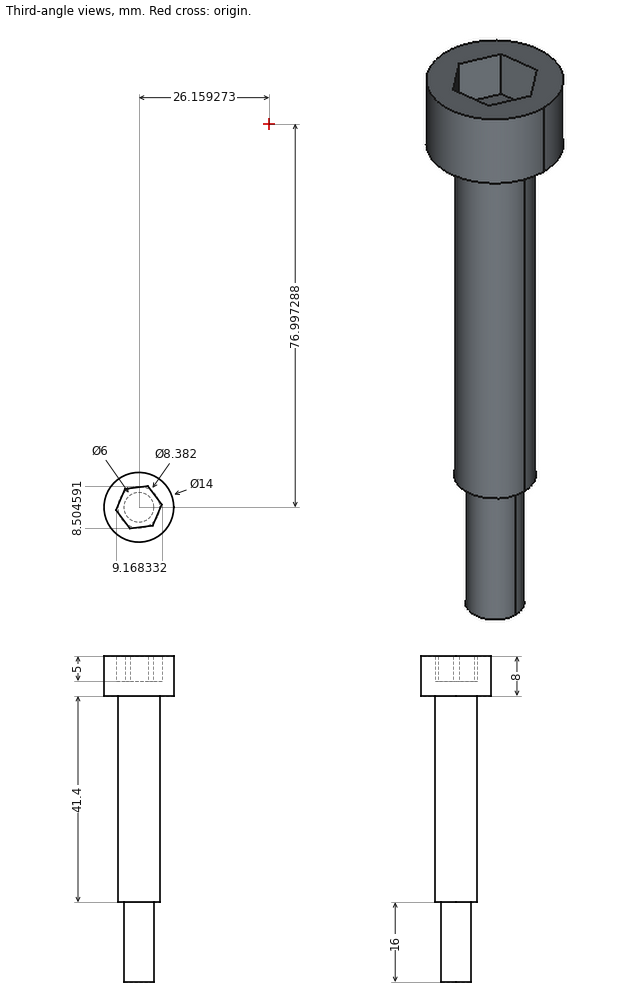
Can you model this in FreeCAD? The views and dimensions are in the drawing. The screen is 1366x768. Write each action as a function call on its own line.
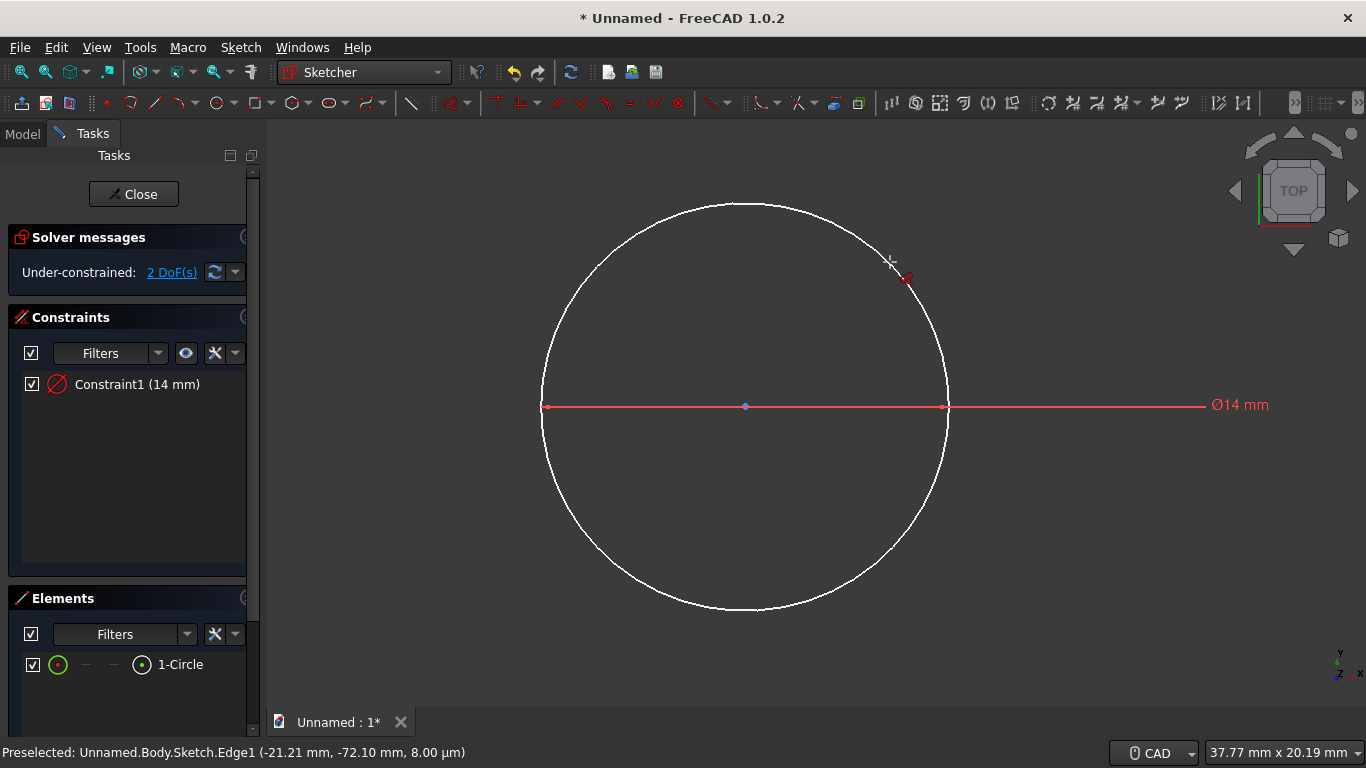
click(745, 407)
click(973, 441)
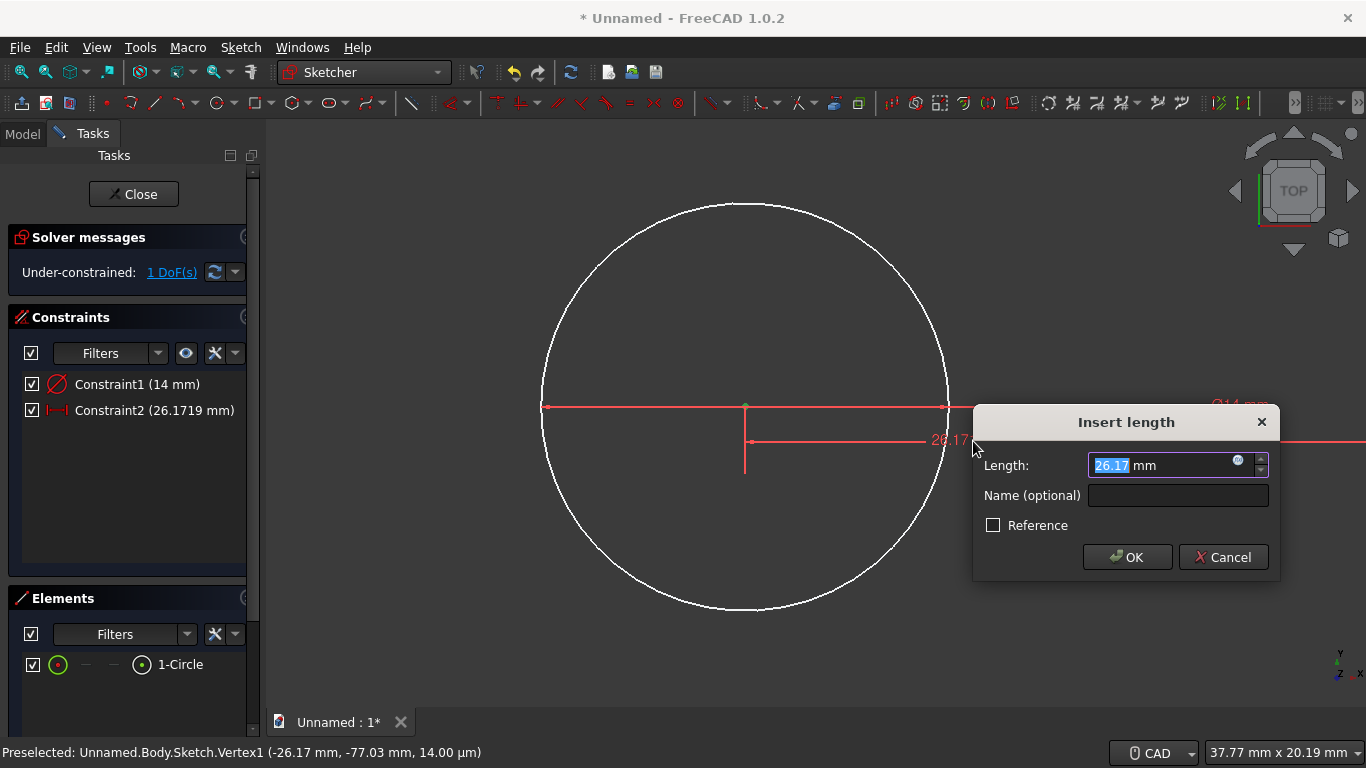
text(26.159273)
key(Return)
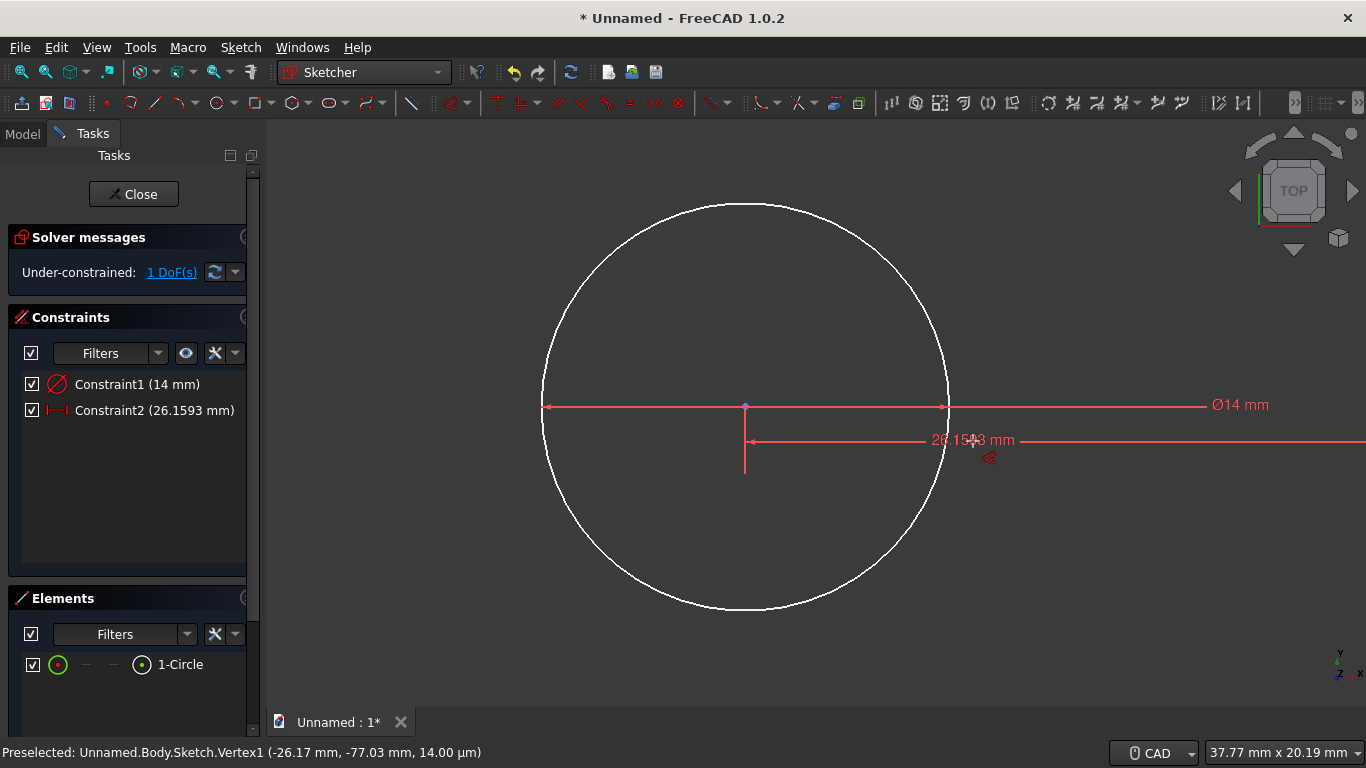
click(745, 407)
click(711, 277)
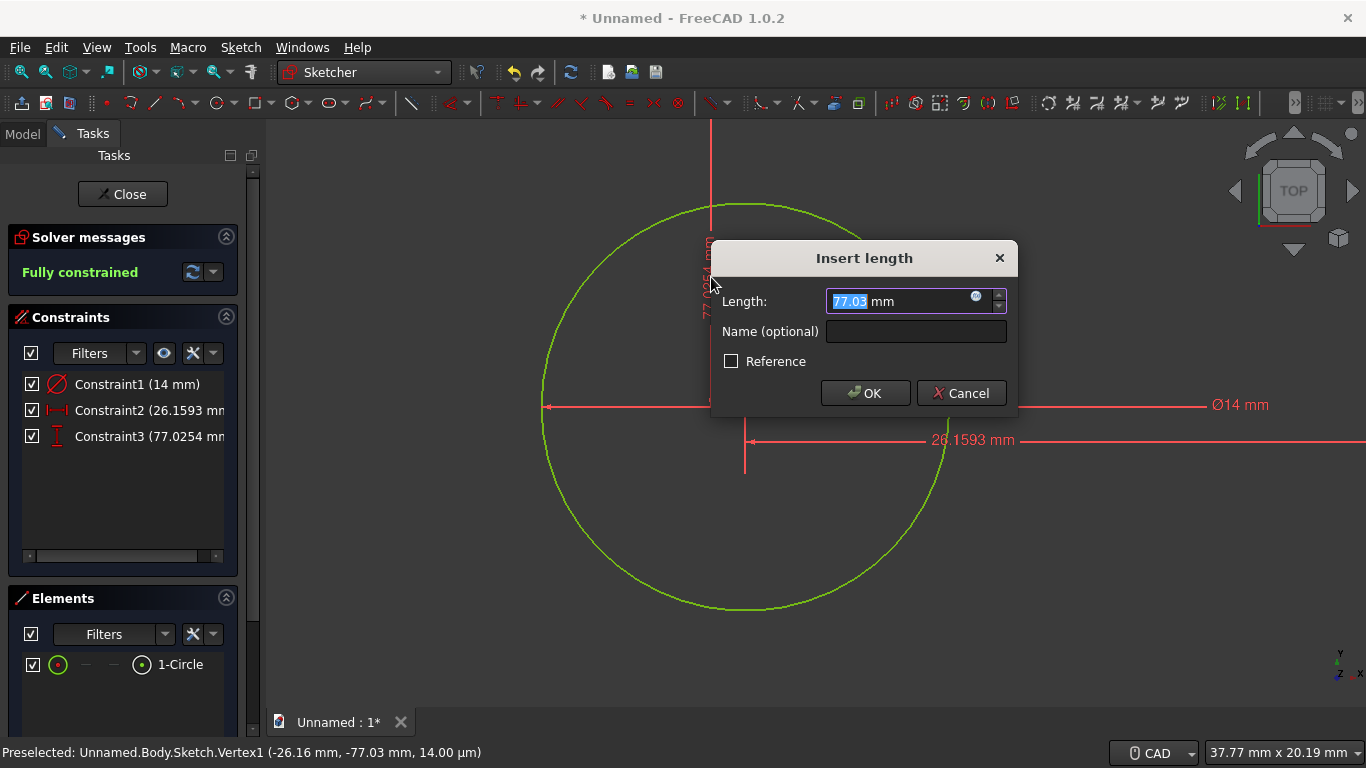
text(76.997288)
key(Return)
key(Escape)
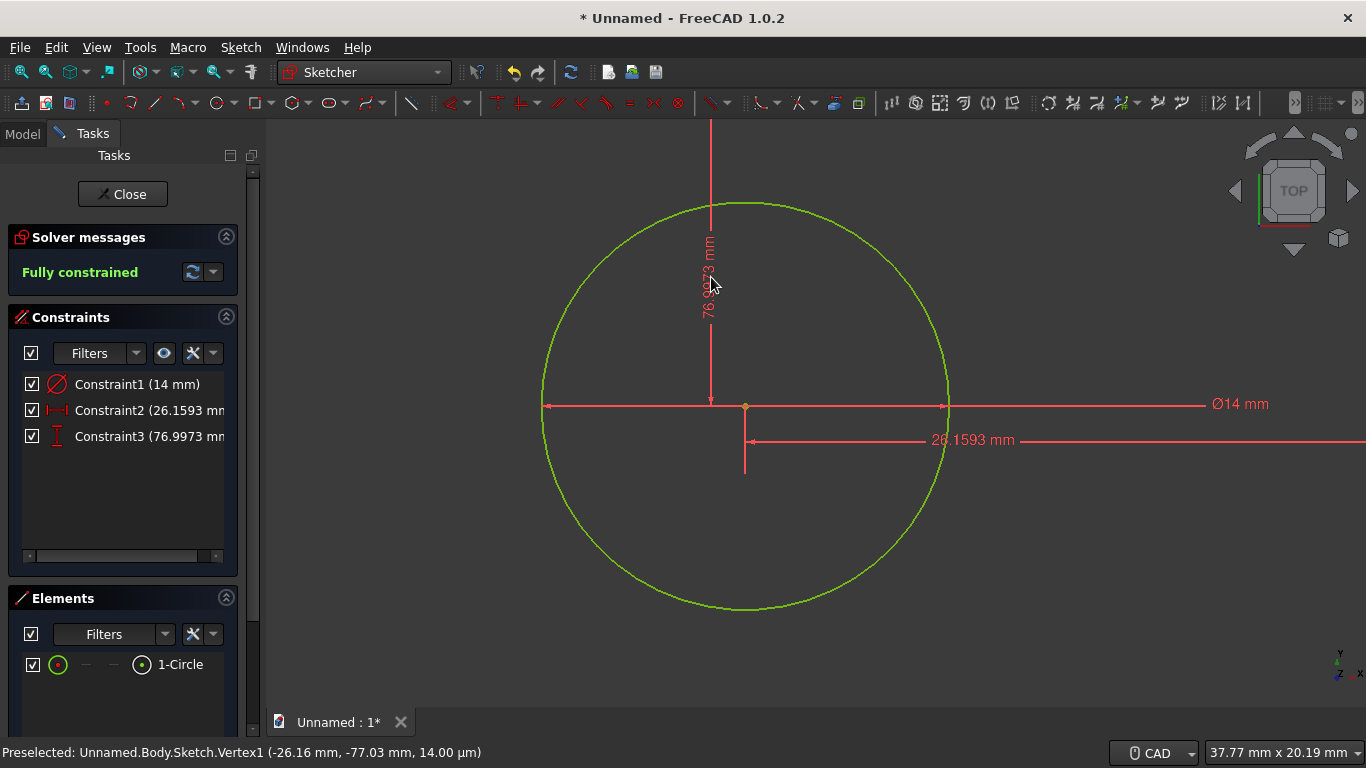
click(123, 194)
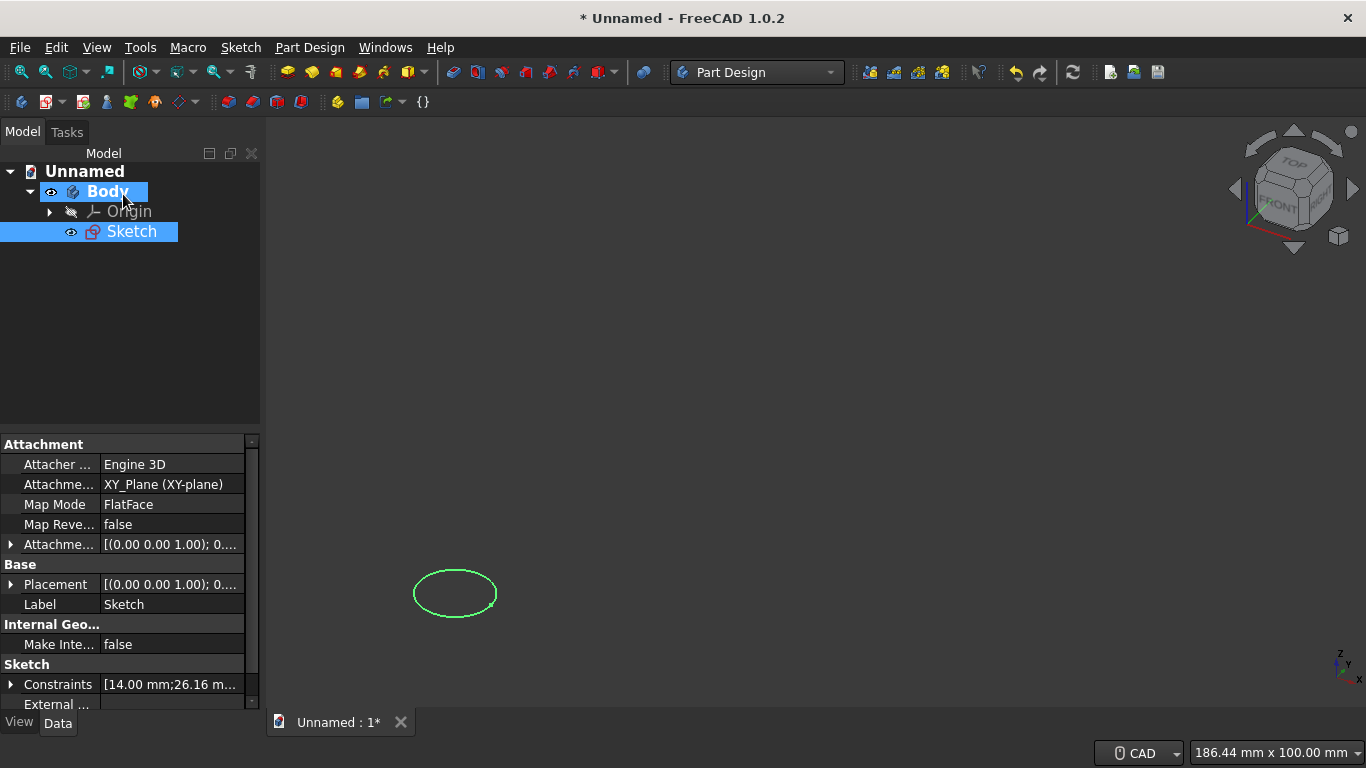
click(288, 72)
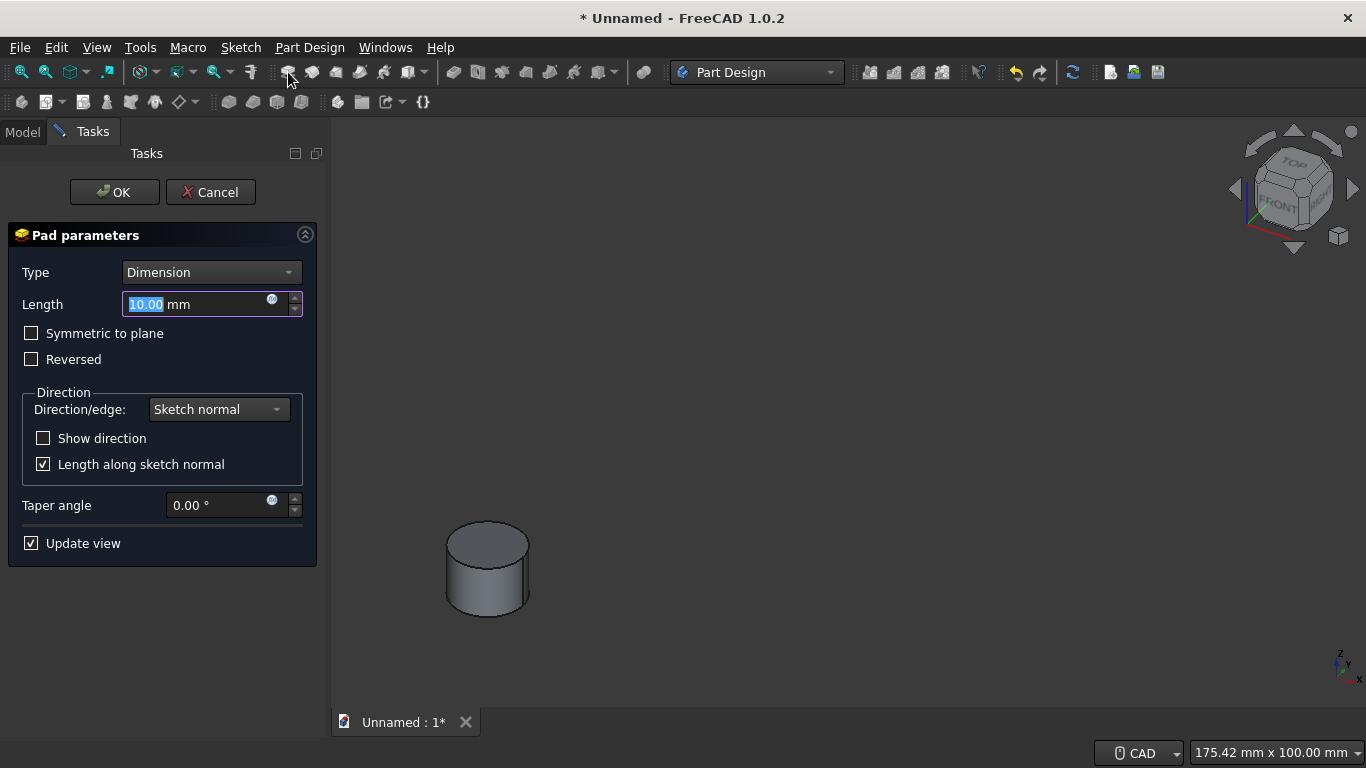
text(8)
key(Tab)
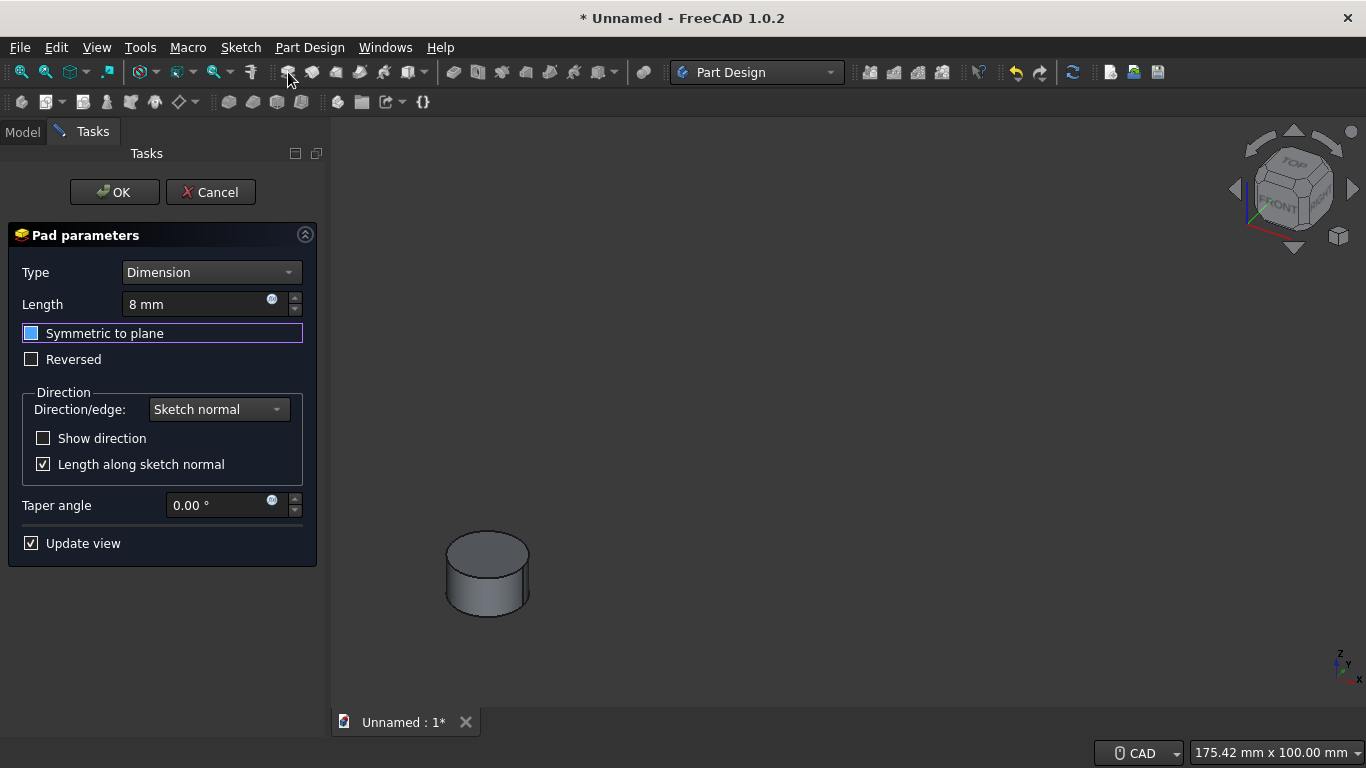
click(115, 192)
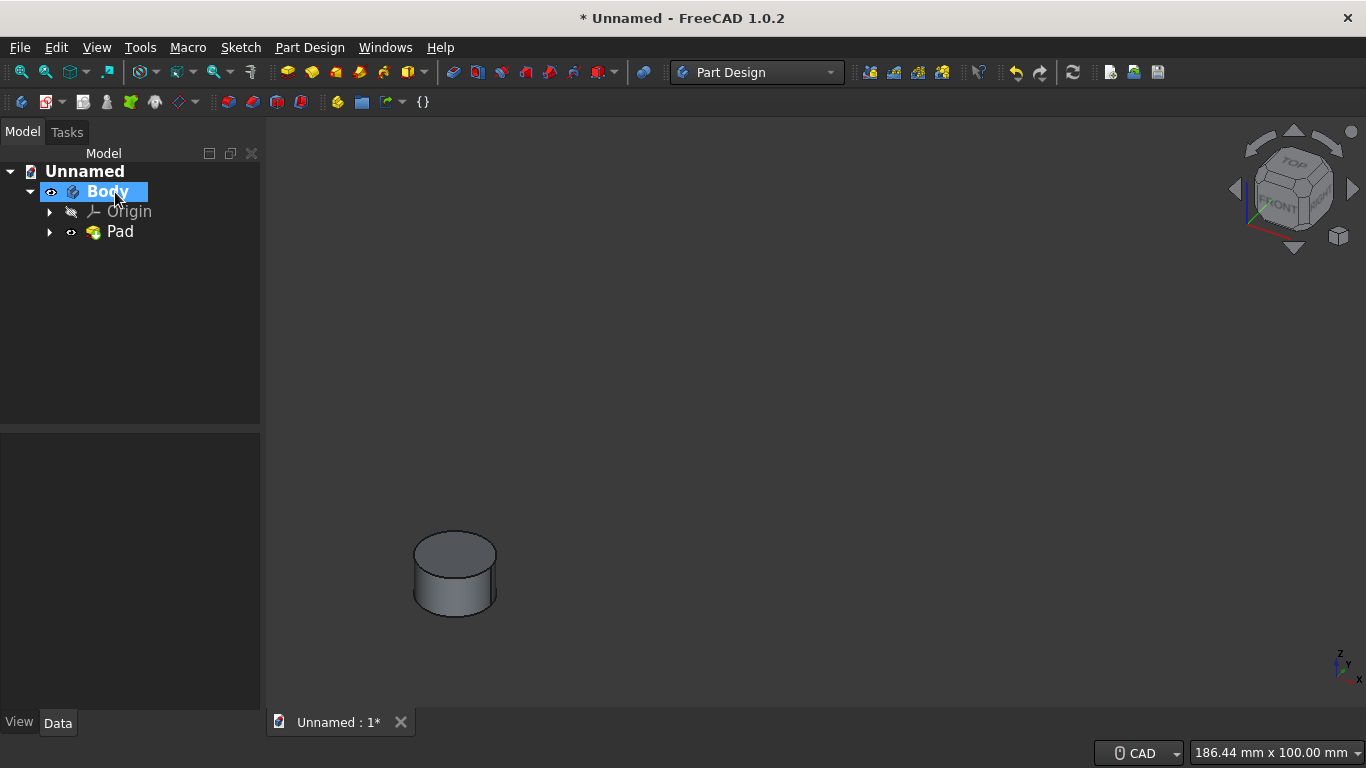
click(22, 72)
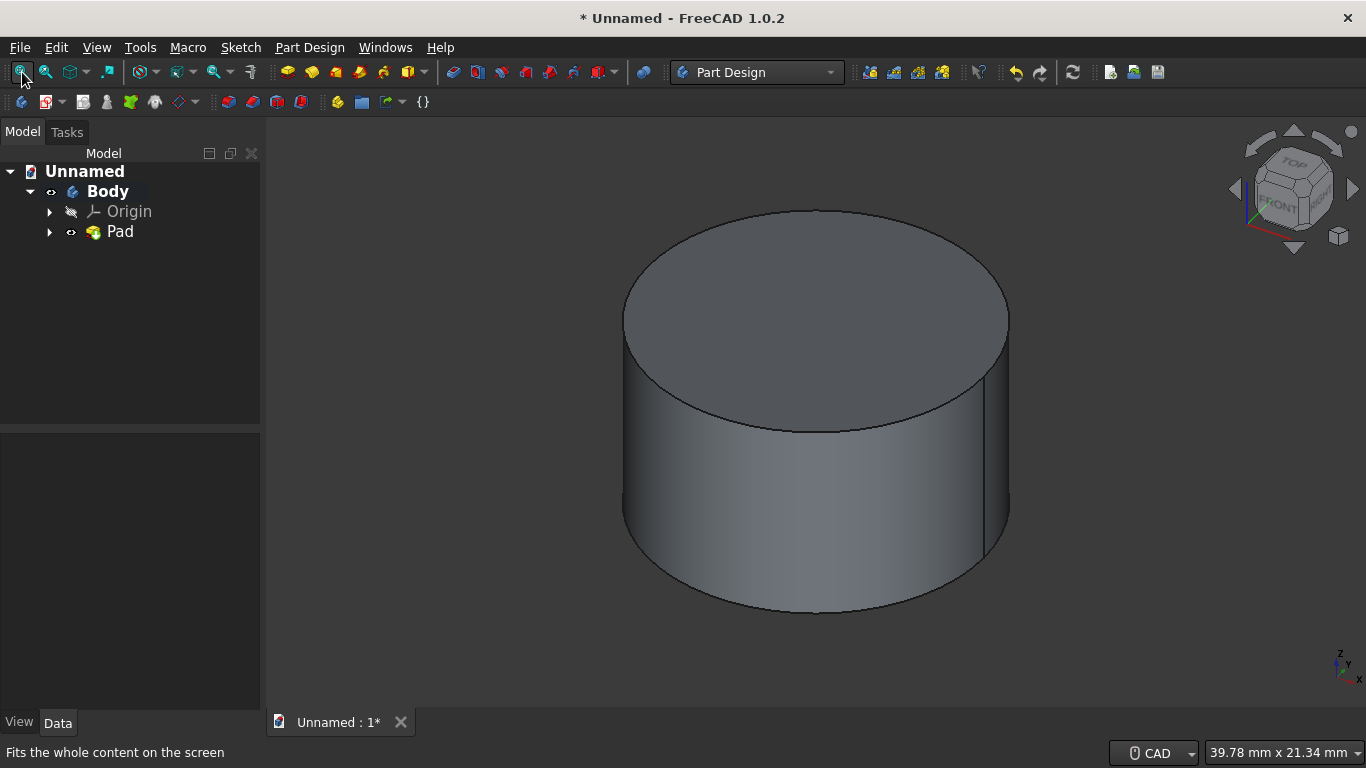
key(5)